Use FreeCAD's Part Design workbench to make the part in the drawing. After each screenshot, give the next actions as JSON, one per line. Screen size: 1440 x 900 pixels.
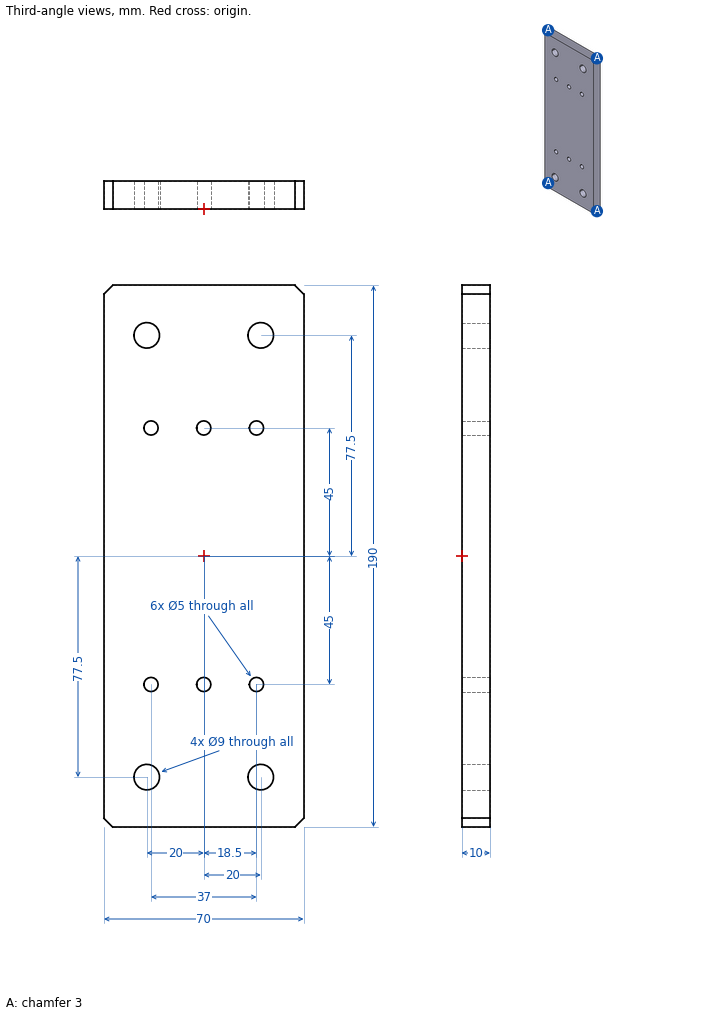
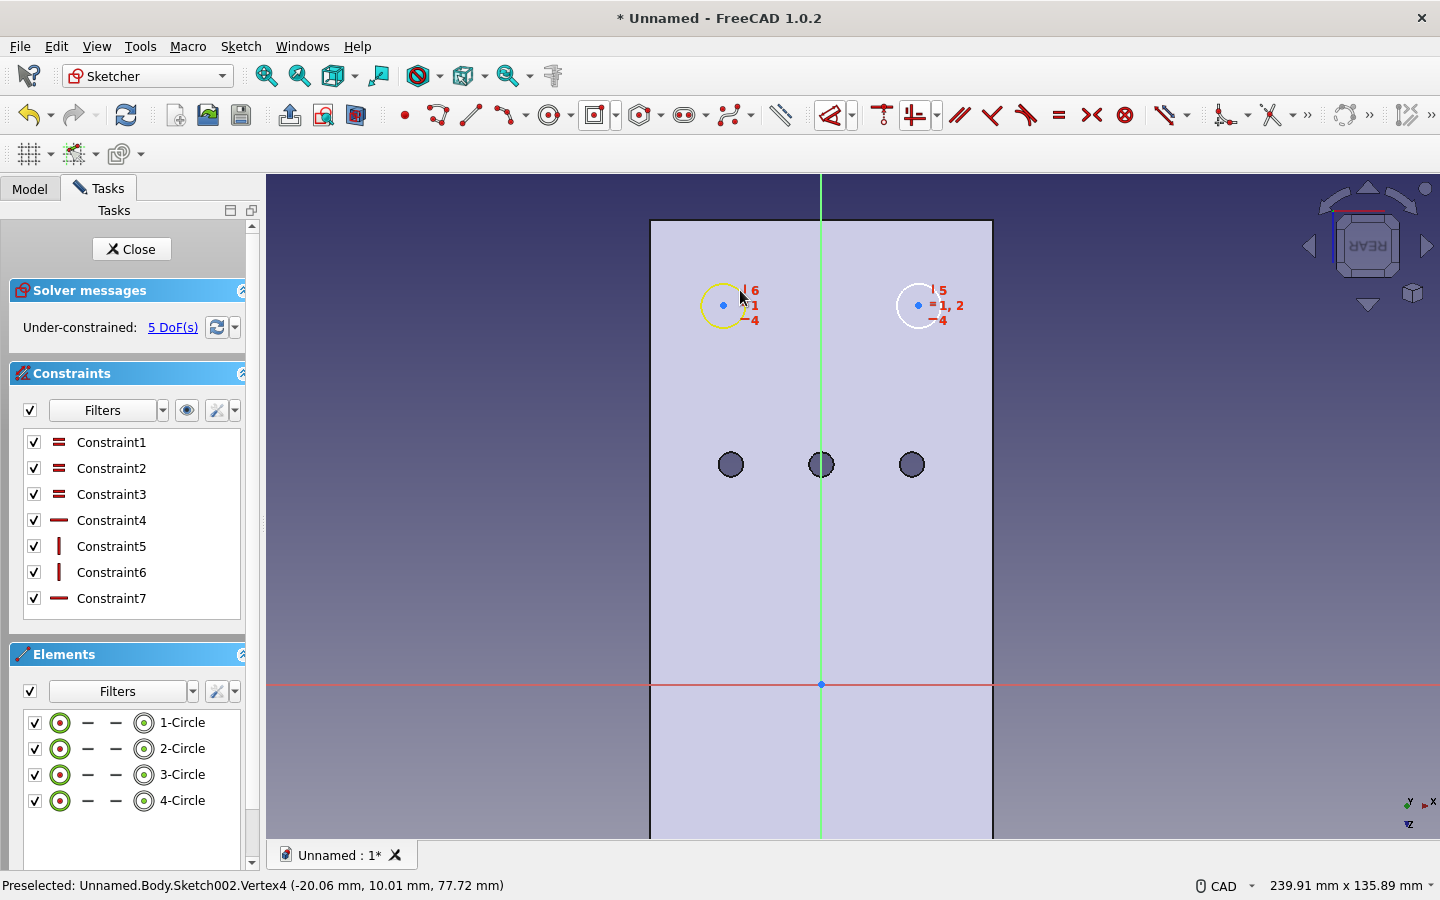
{"action": "left_click", "coordinate": [739, 290]}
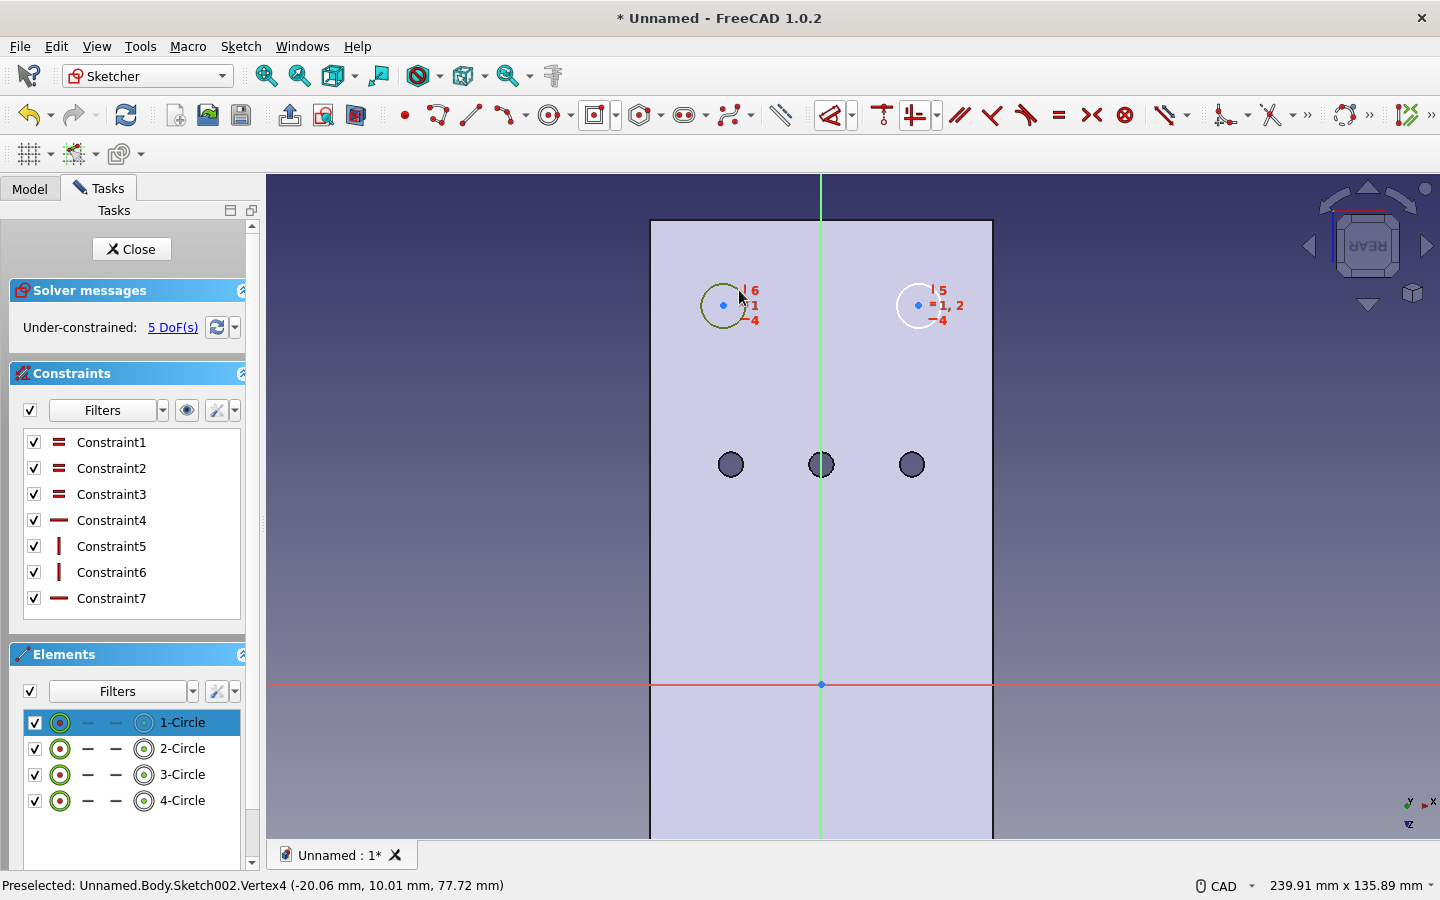
{"action": "left_click", "coordinate": [852, 116]}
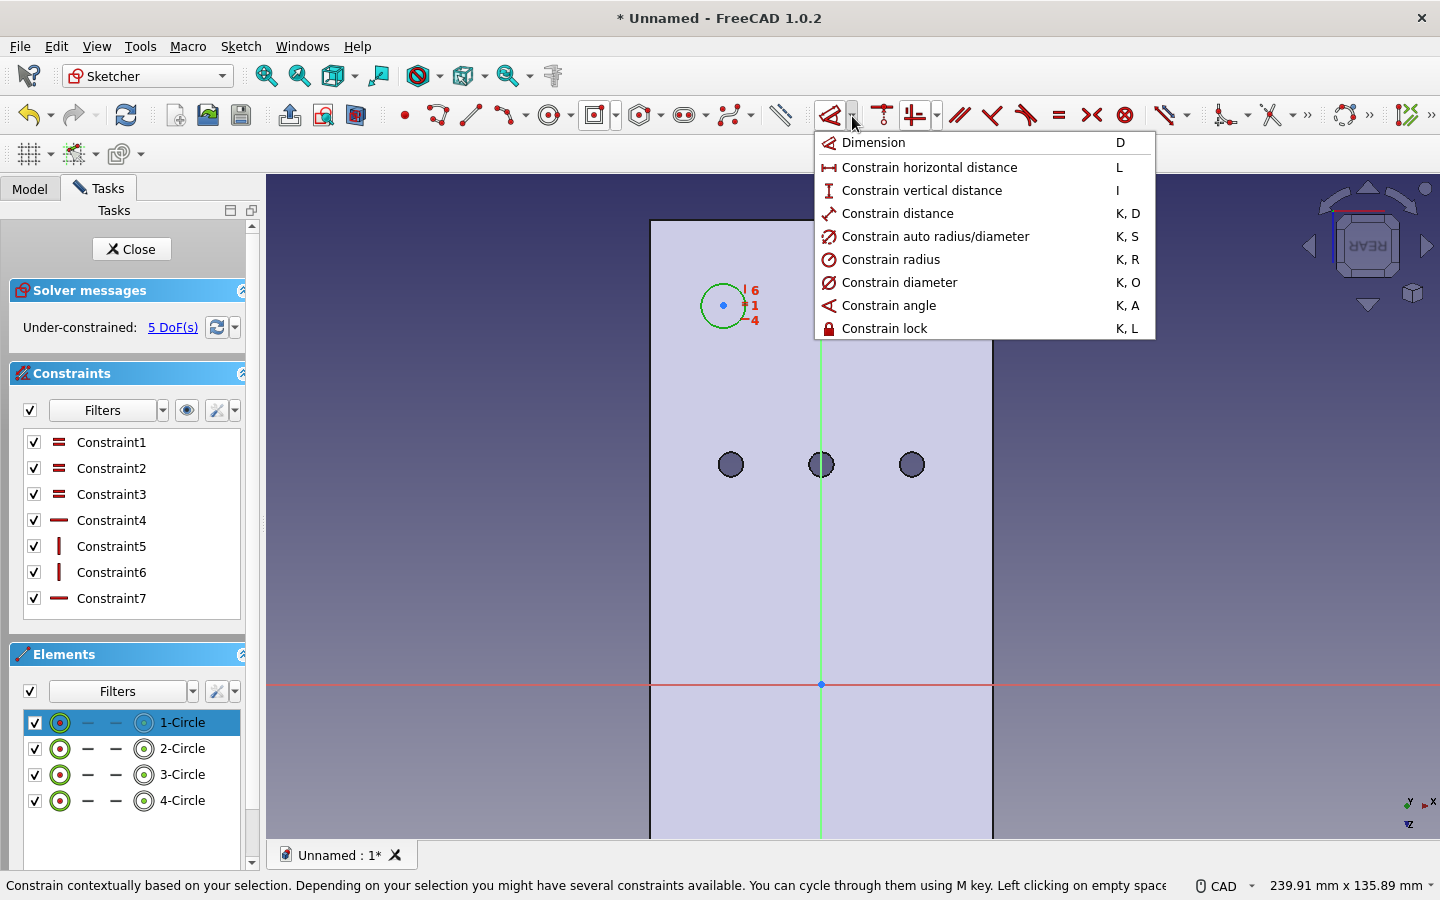
{"action": "left_click", "coordinate": [985, 282]}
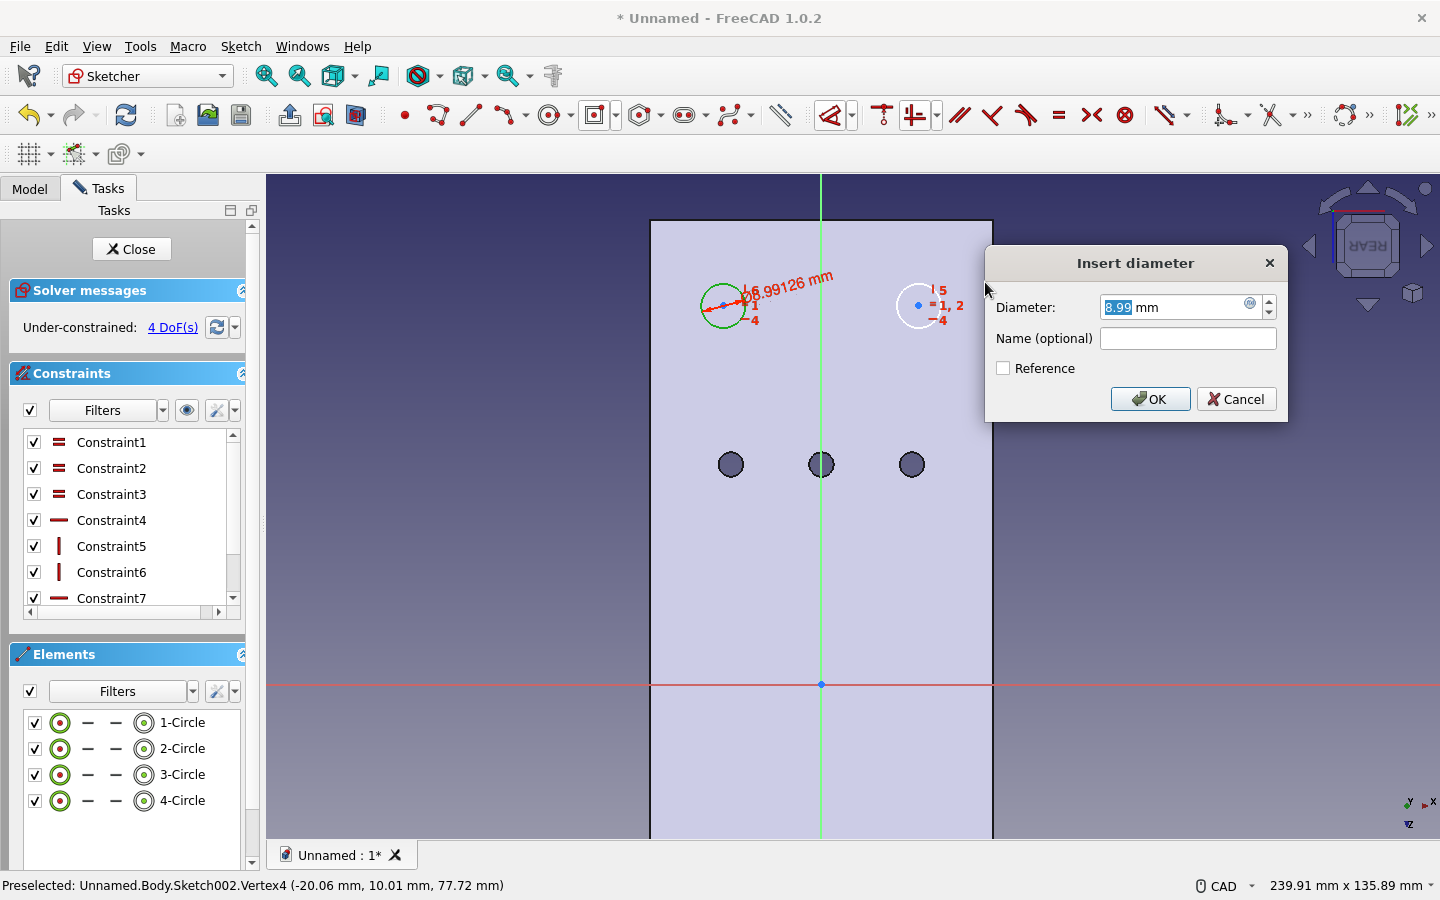
{"action": "type", "text": "9"}
{"action": "key", "text": "Return"}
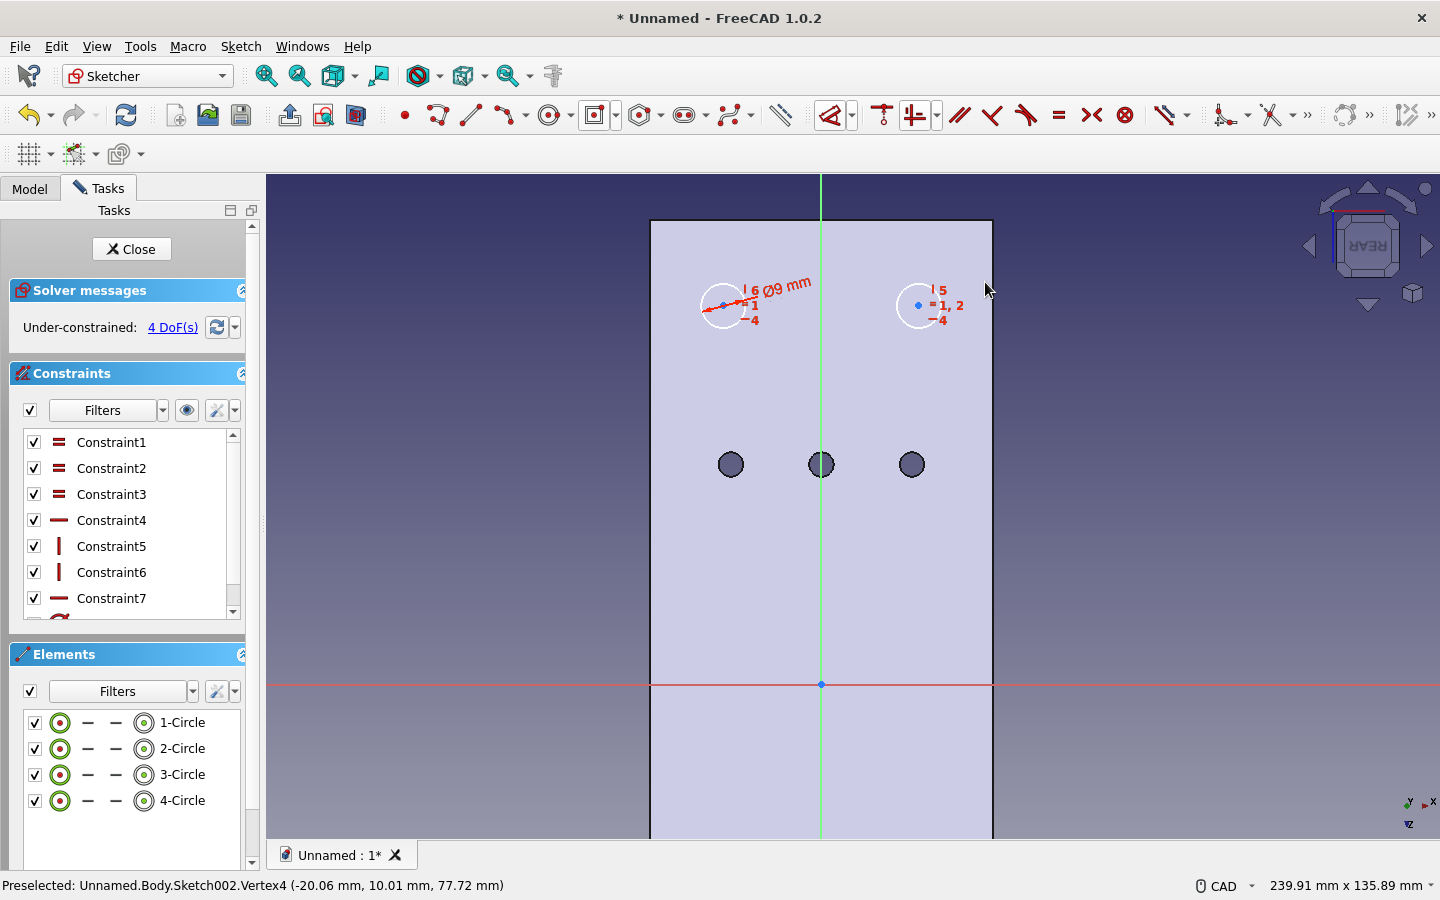
{"action": "left_click", "coordinate": [723, 306]}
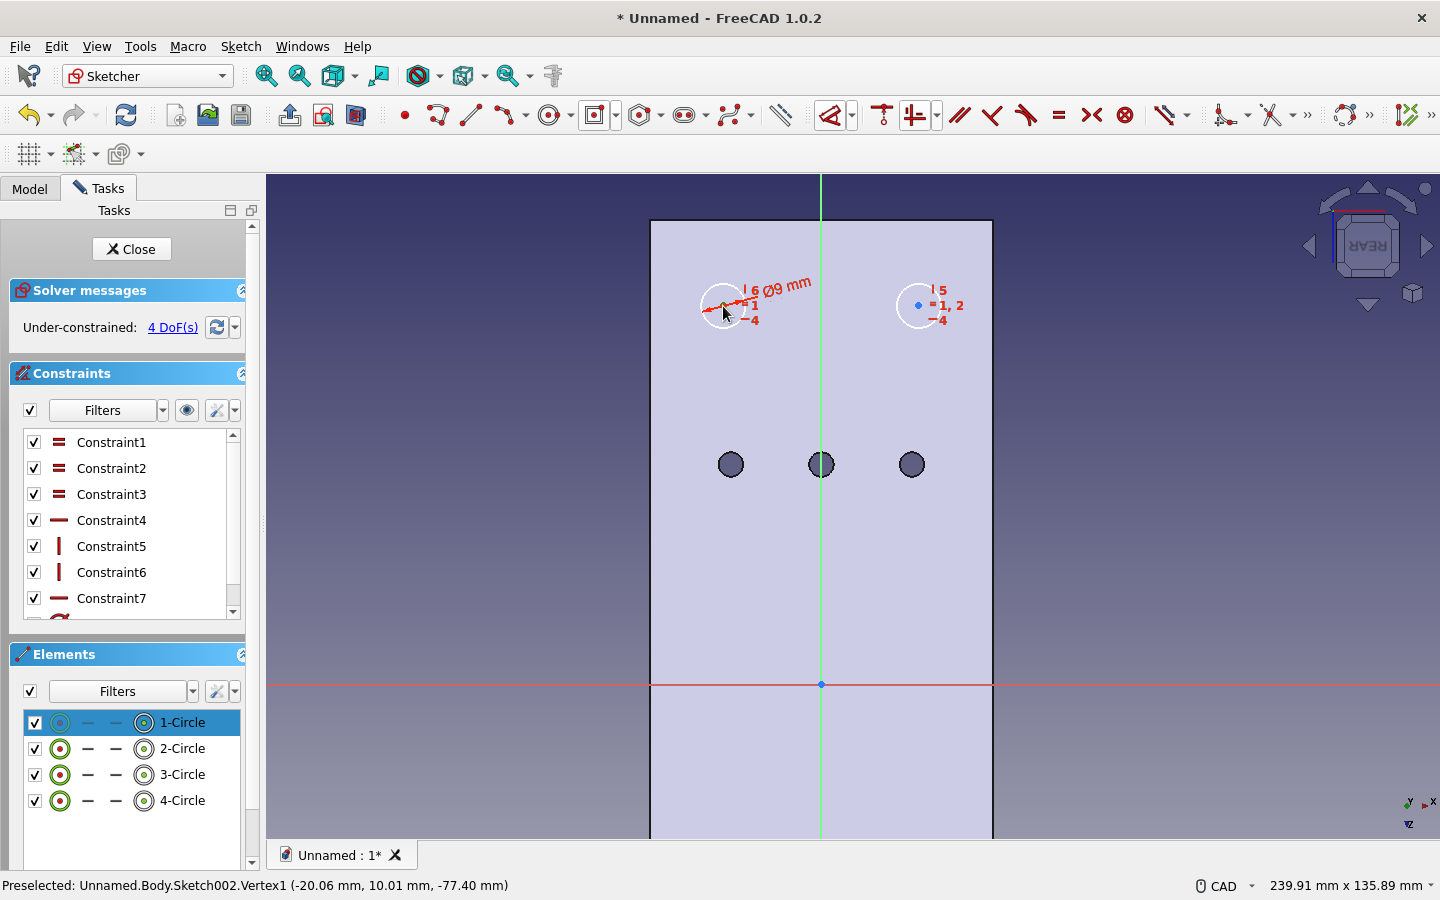
{"action": "key", "text": "l"}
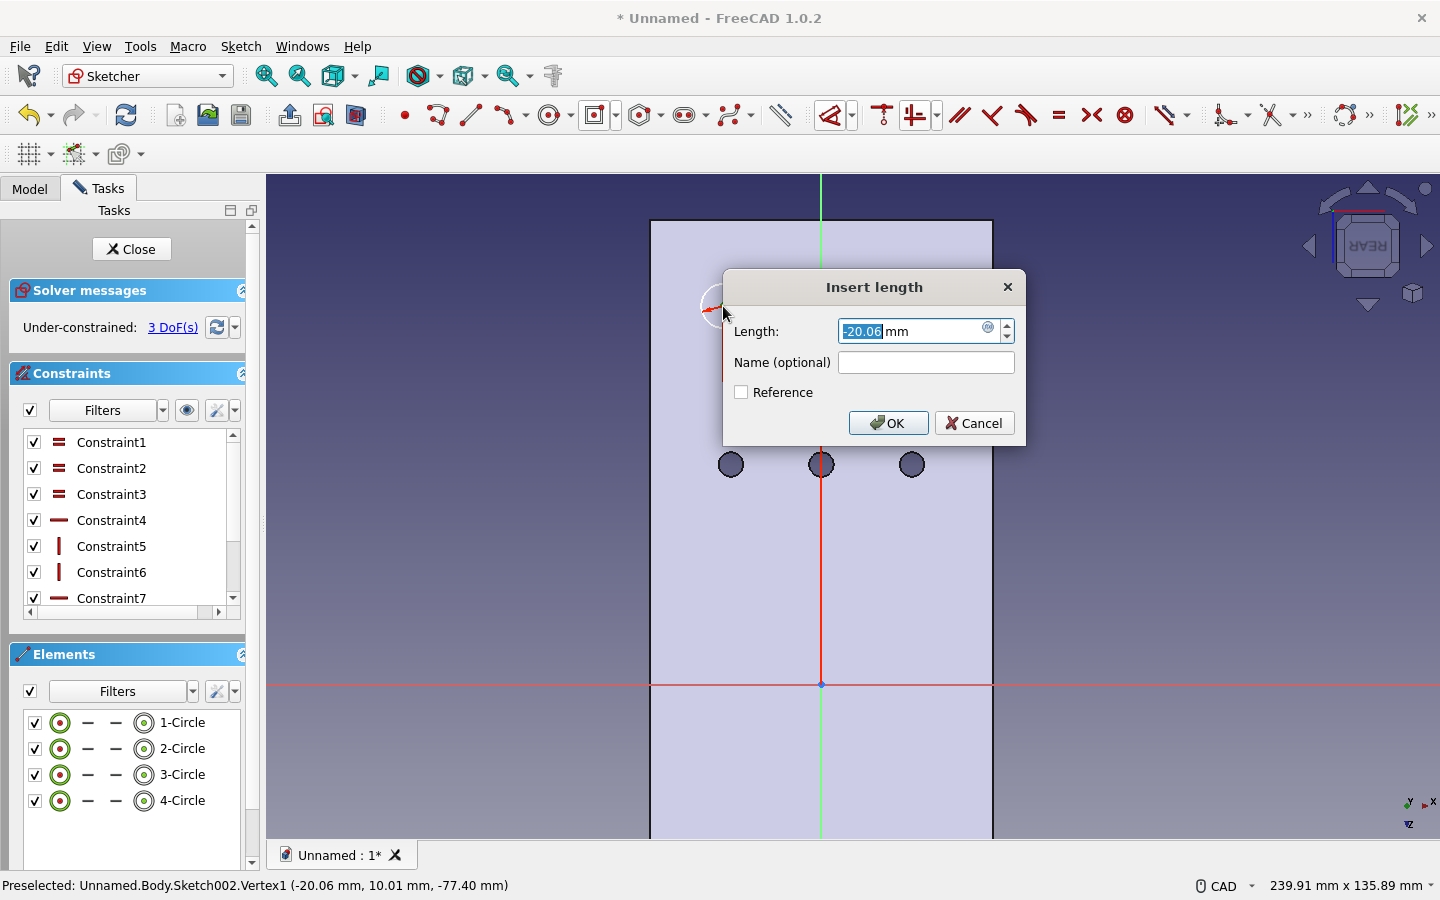
{"action": "type", "text": "-20"}
{"action": "key", "text": "Return"}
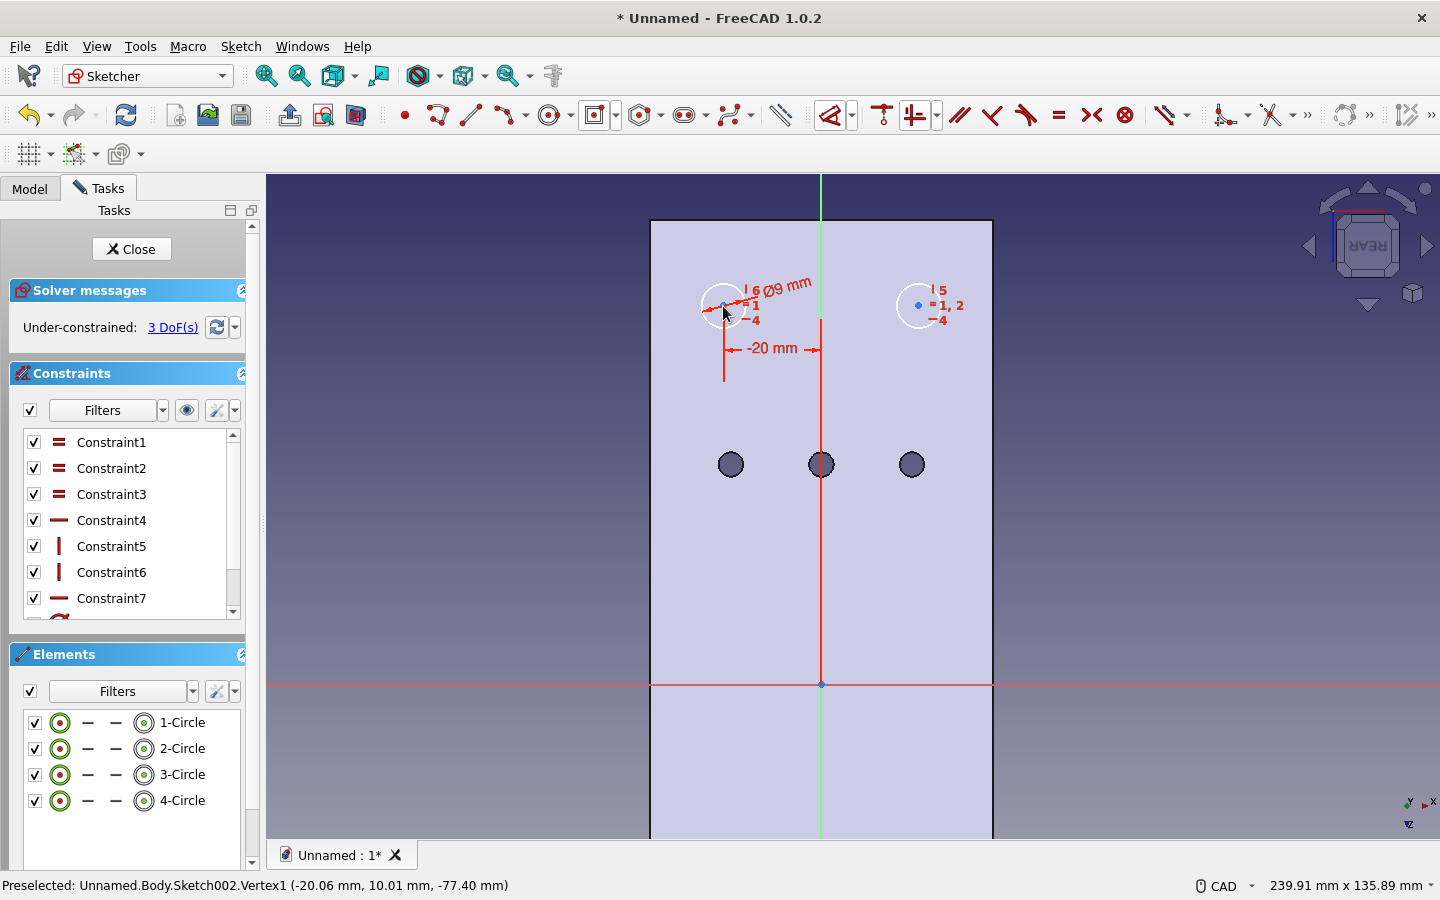
{"action": "left_click", "coordinate": [919, 306]}